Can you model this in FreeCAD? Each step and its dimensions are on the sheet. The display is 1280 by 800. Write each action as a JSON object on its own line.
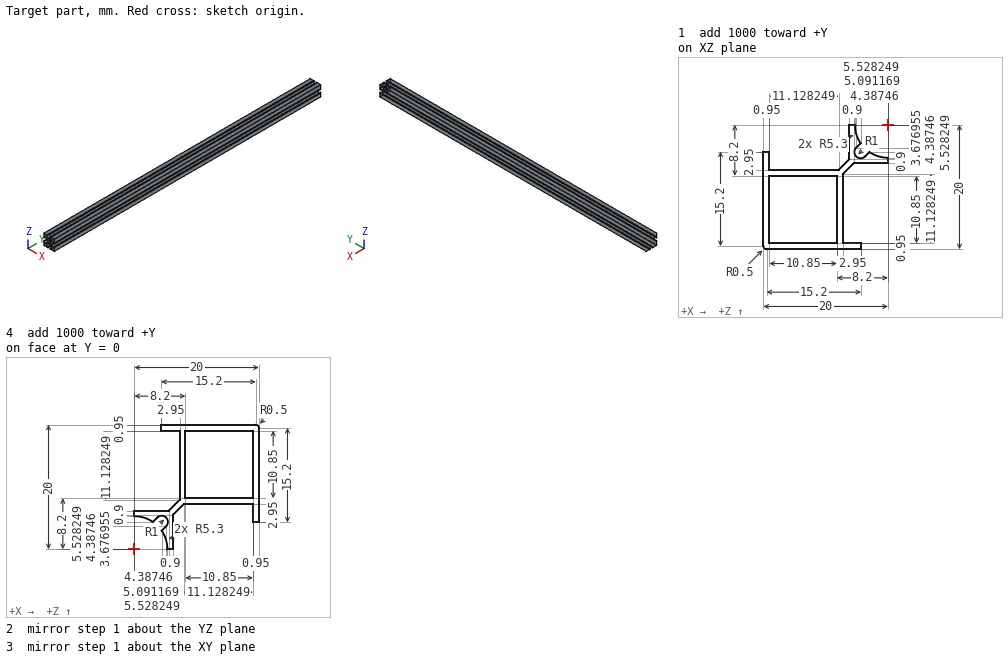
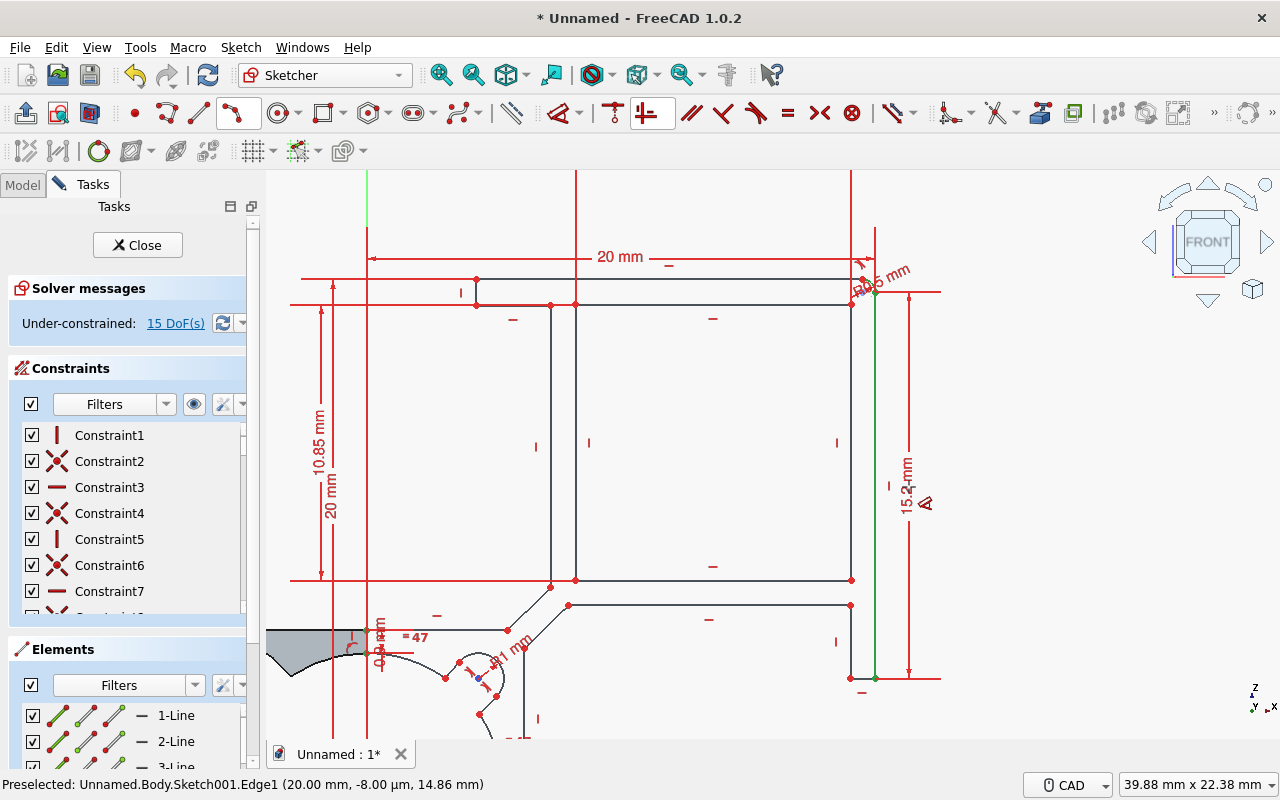
{"action": "scroll", "coordinate": [865, 679], "scroll_direction": "up", "scroll_amount": 3}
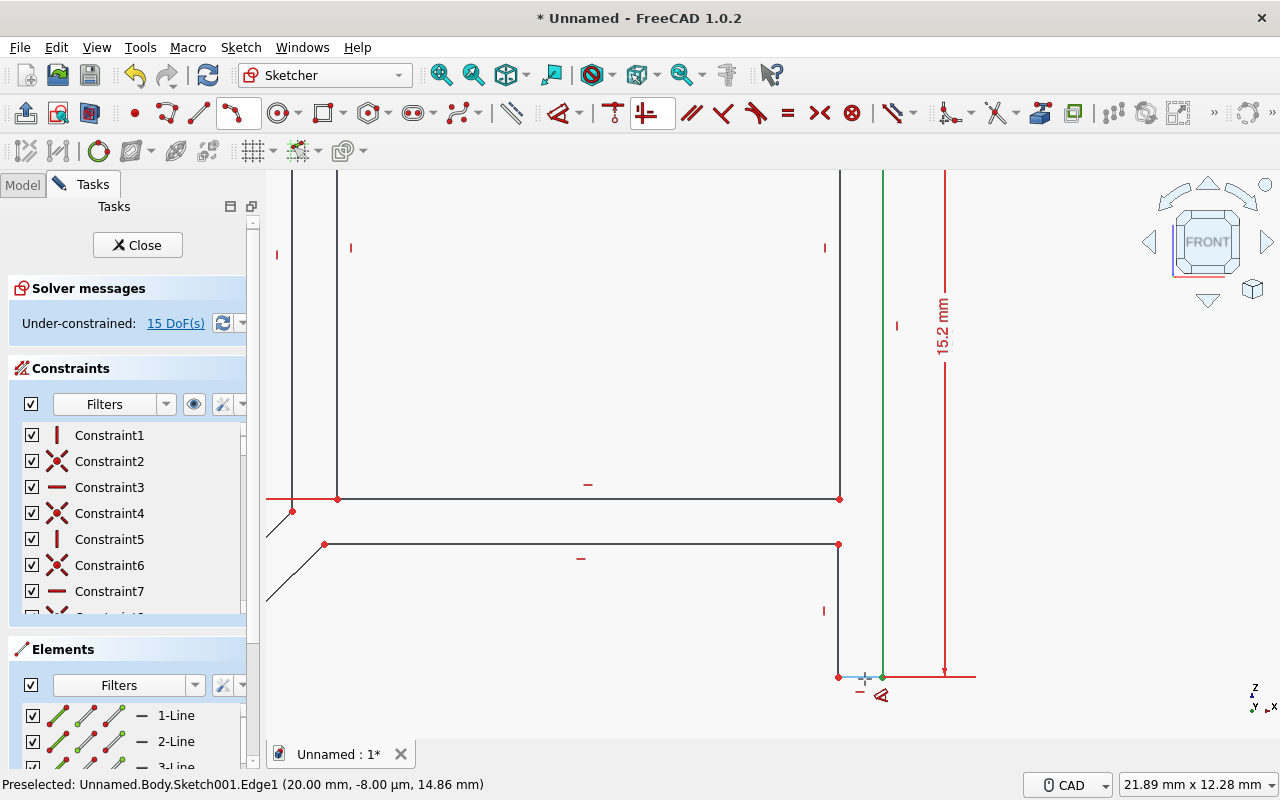
{"action": "left_click", "coordinate": [865, 677]}
{"action": "left_click", "coordinate": [861, 643]}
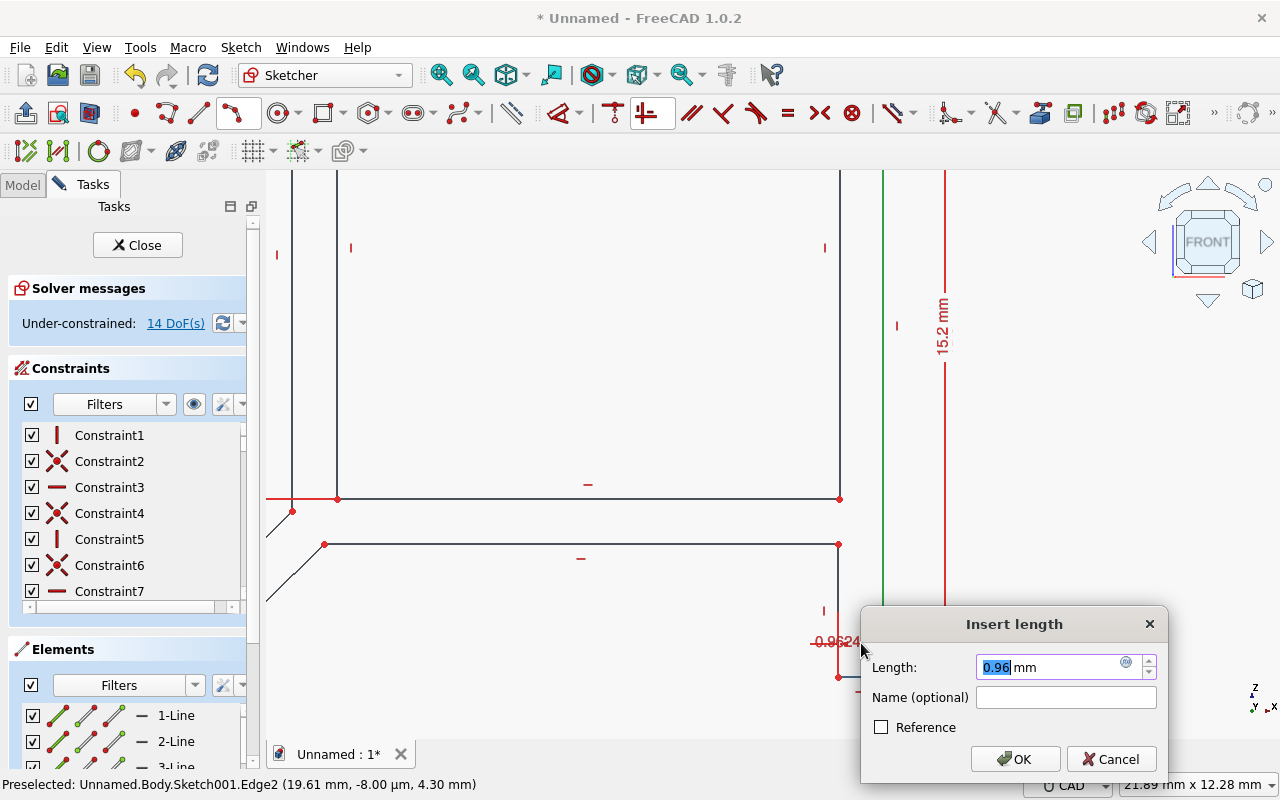
{"action": "type", "text": "0.95"}
{"action": "key", "text": "Return"}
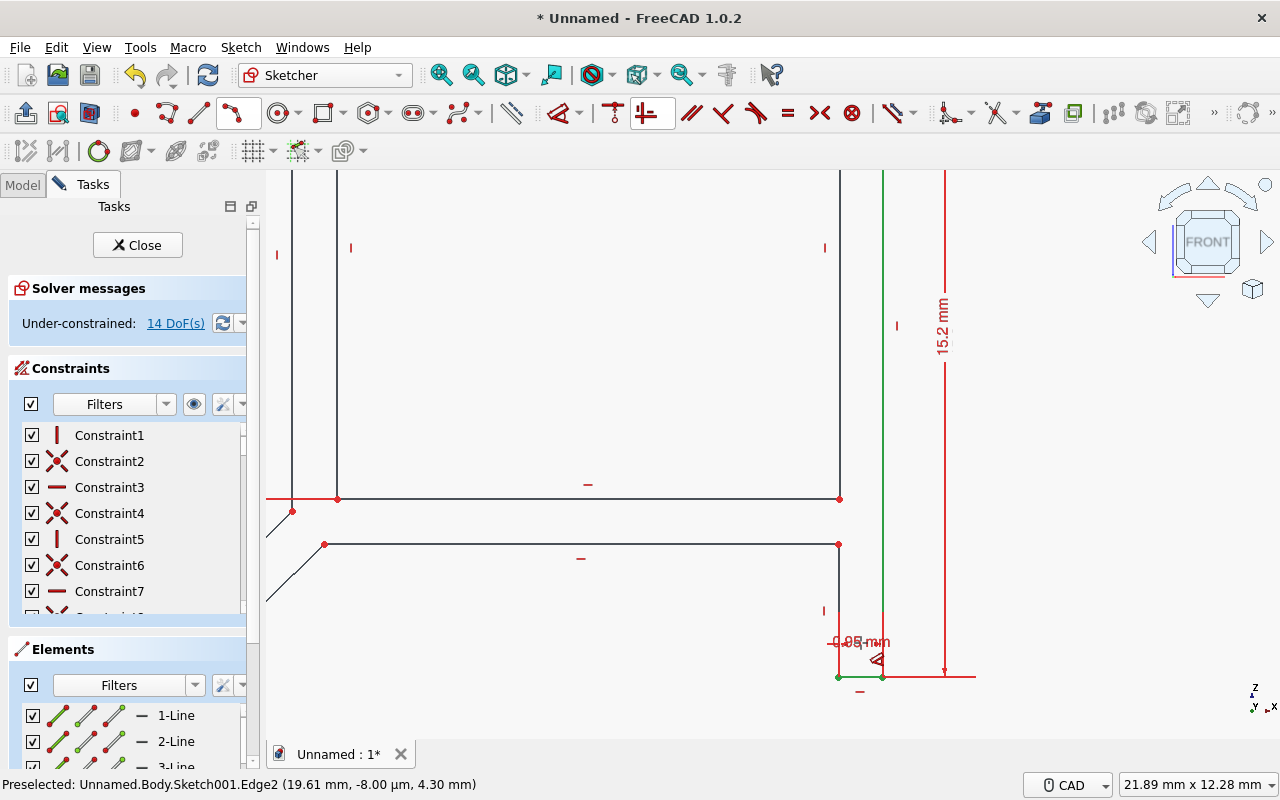
{"action": "scroll", "coordinate": [870, 478], "scroll_direction": "down", "scroll_amount": 5}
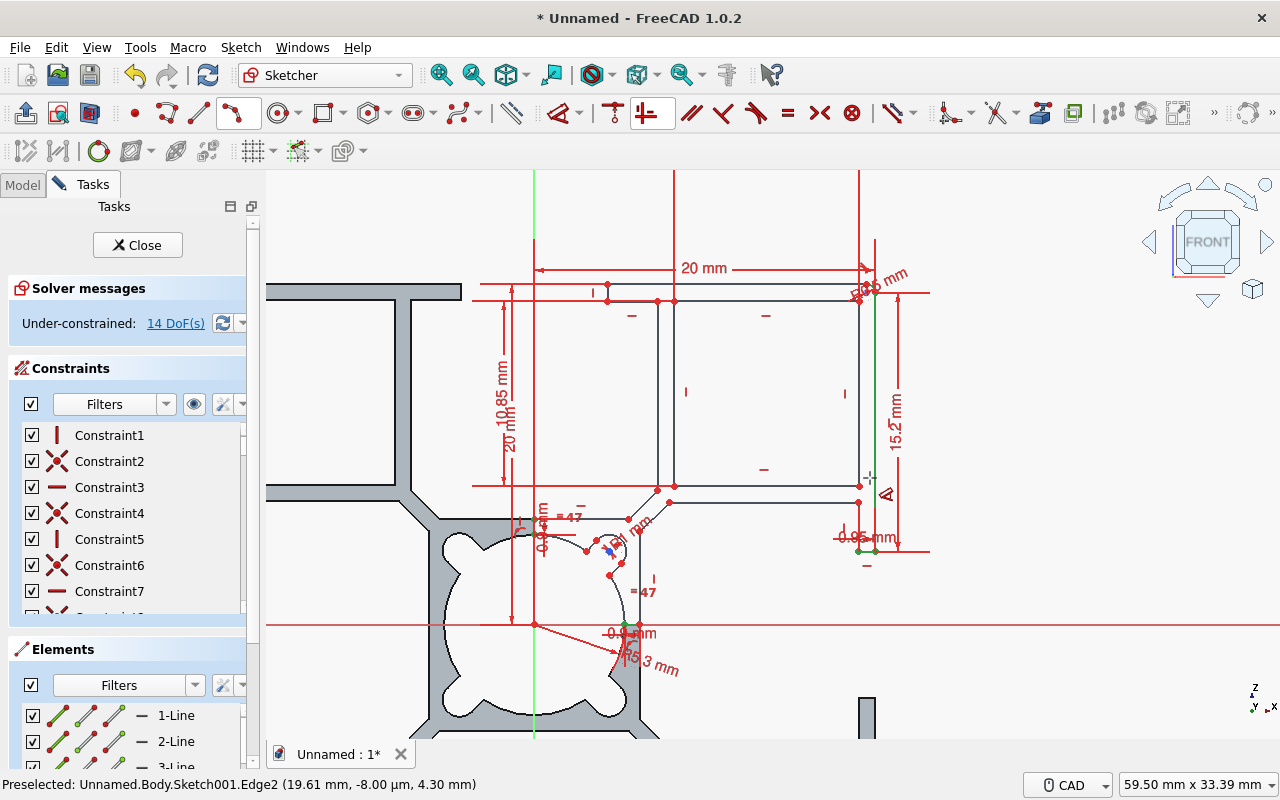
{"action": "left_click", "coordinate": [859, 537]}
{"action": "left_click", "coordinate": [893, 516]}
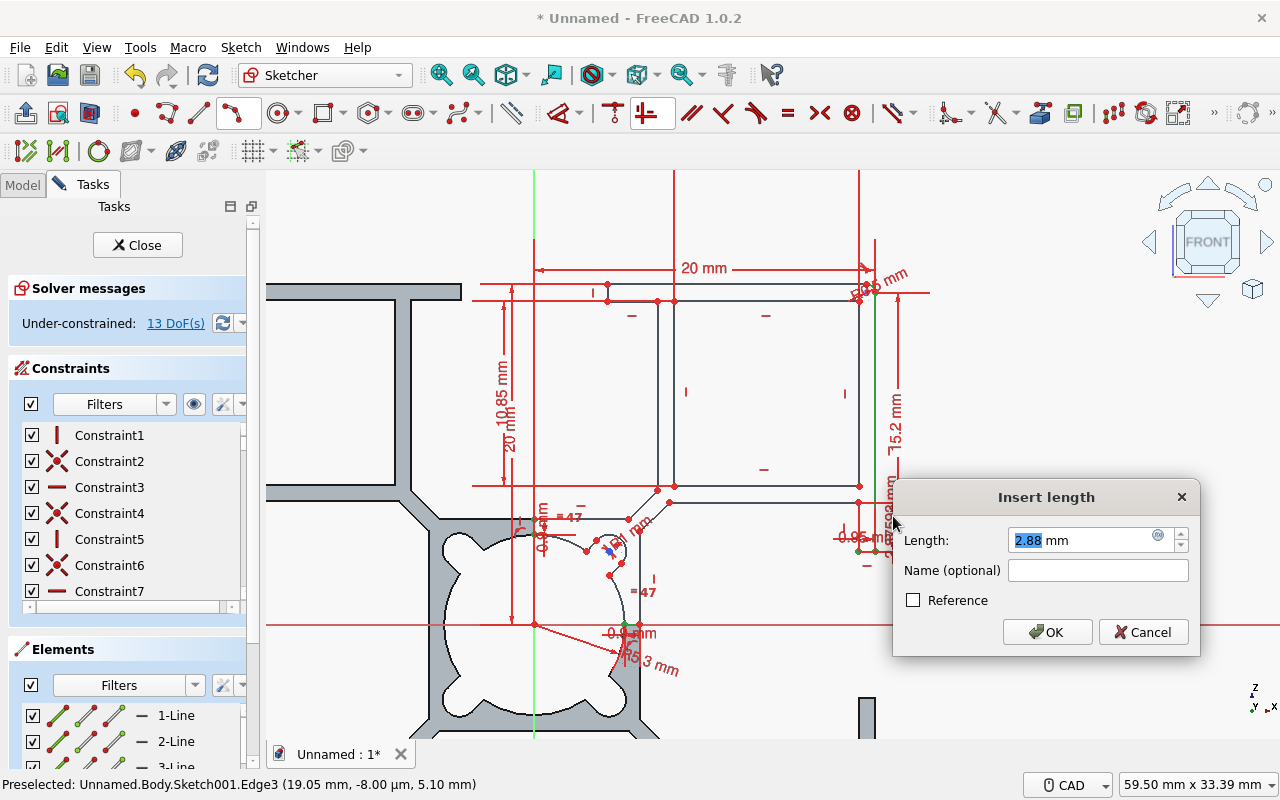
{"action": "type", "text": "2.95"}
{"action": "key", "text": "Return"}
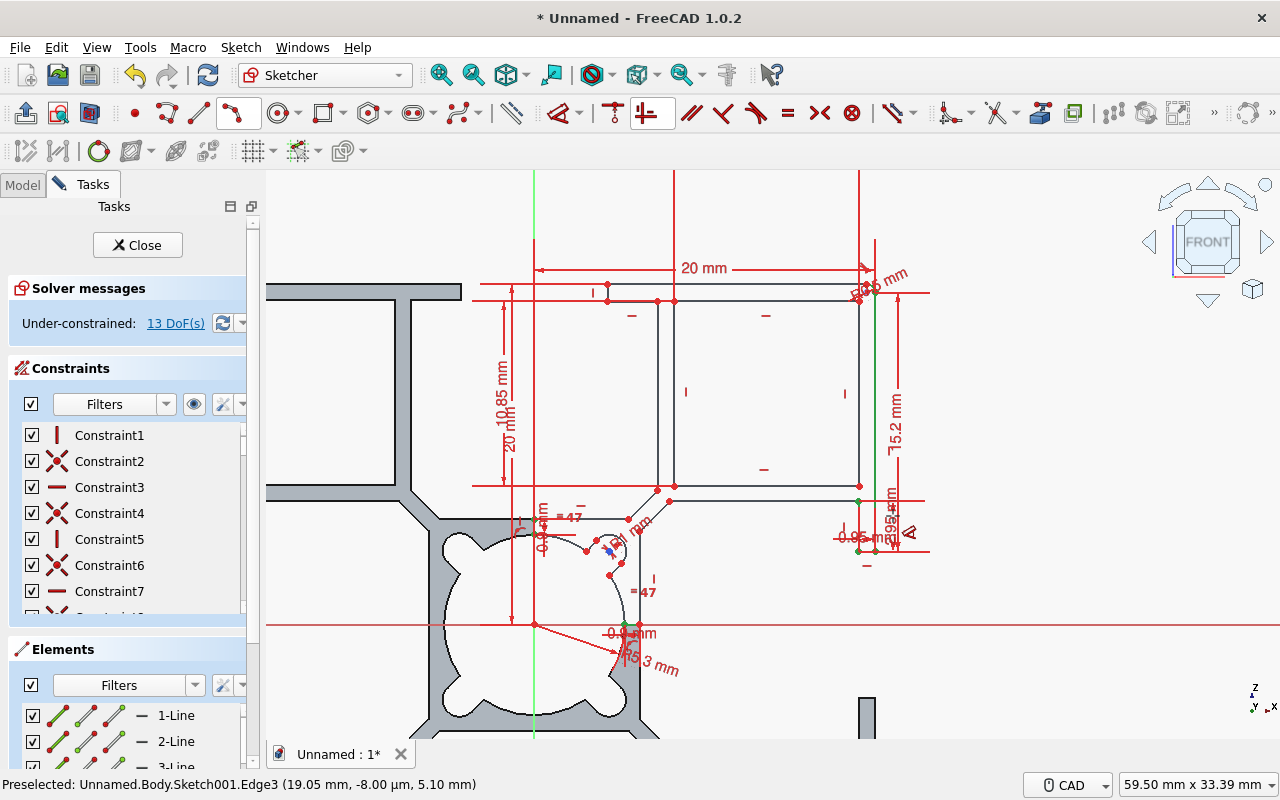
{"action": "left_click", "coordinate": [643, 302]}
{"action": "left_click", "coordinate": [633, 268]}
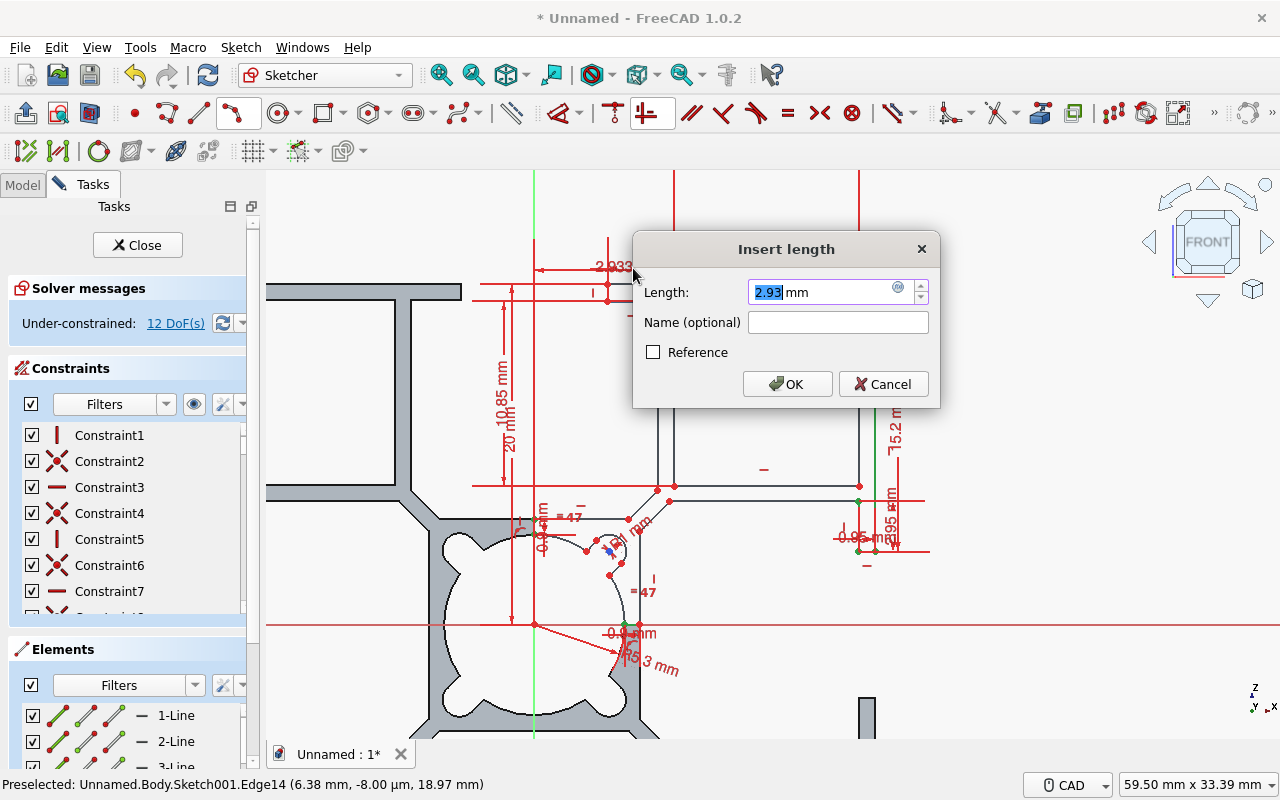
{"action": "type", "text": "2.95"}
{"action": "key", "text": "Return"}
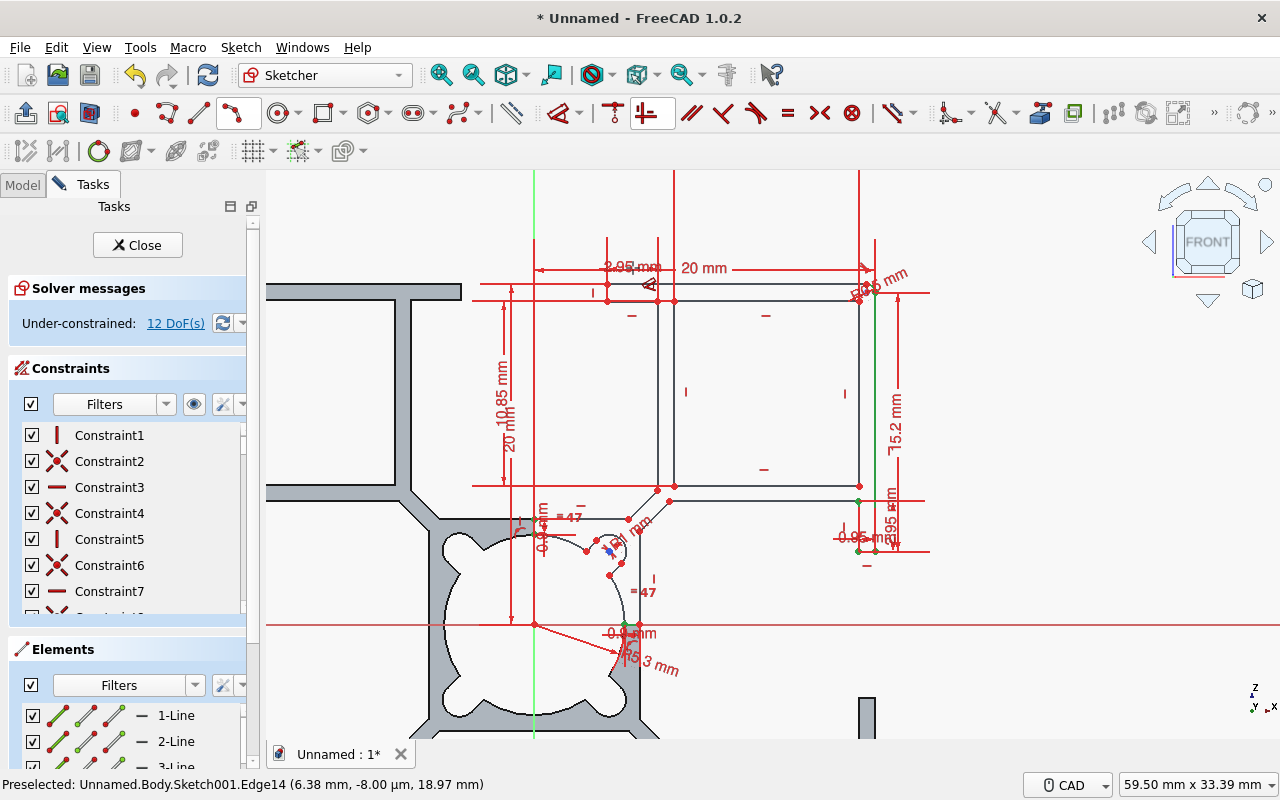
{"action": "scroll", "coordinate": [607, 293], "scroll_direction": "up", "scroll_amount": 5}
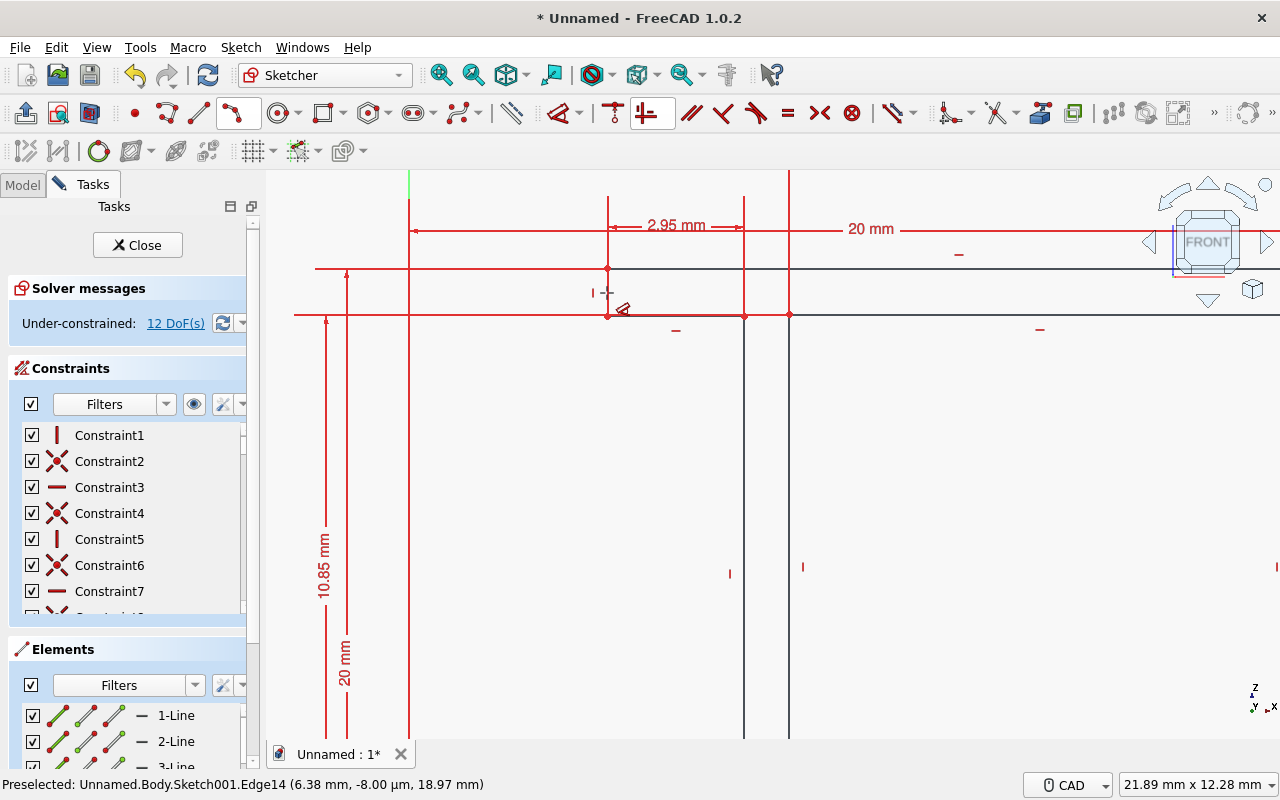
{"action": "left_click", "coordinate": [608, 292]}
{"action": "left_click", "coordinate": [574, 292]}